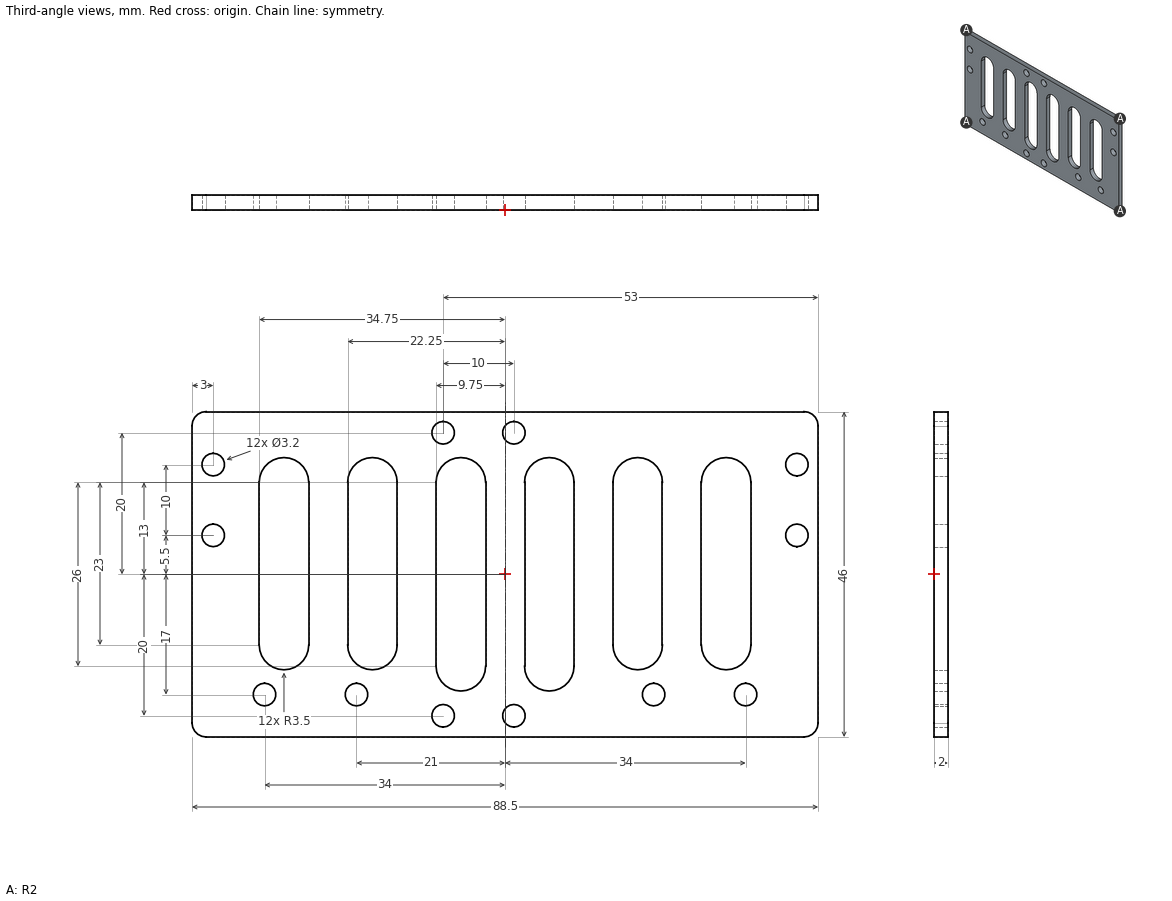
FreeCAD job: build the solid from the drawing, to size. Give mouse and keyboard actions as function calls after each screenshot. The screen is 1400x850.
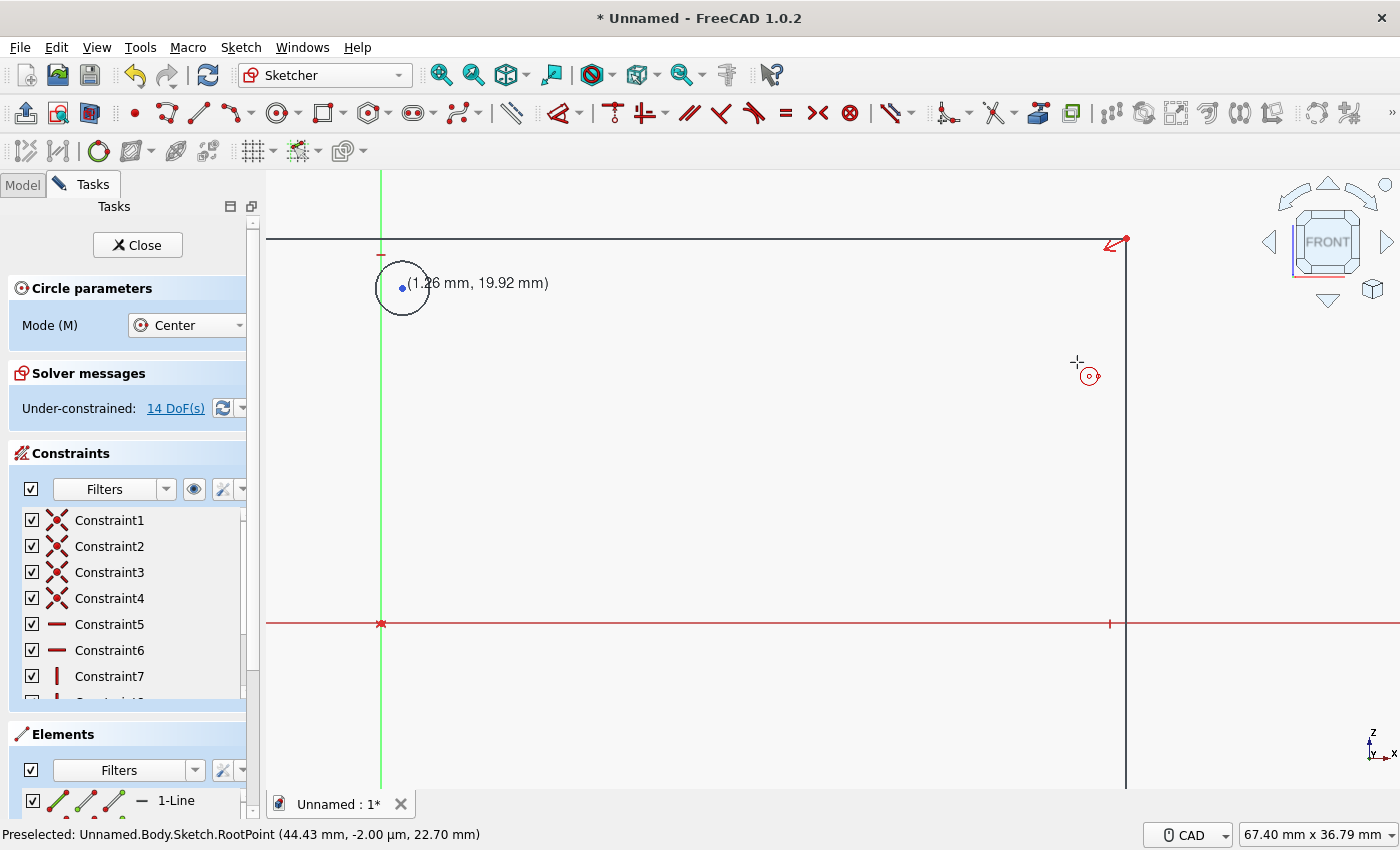
click(1075, 363)
click(1095, 344)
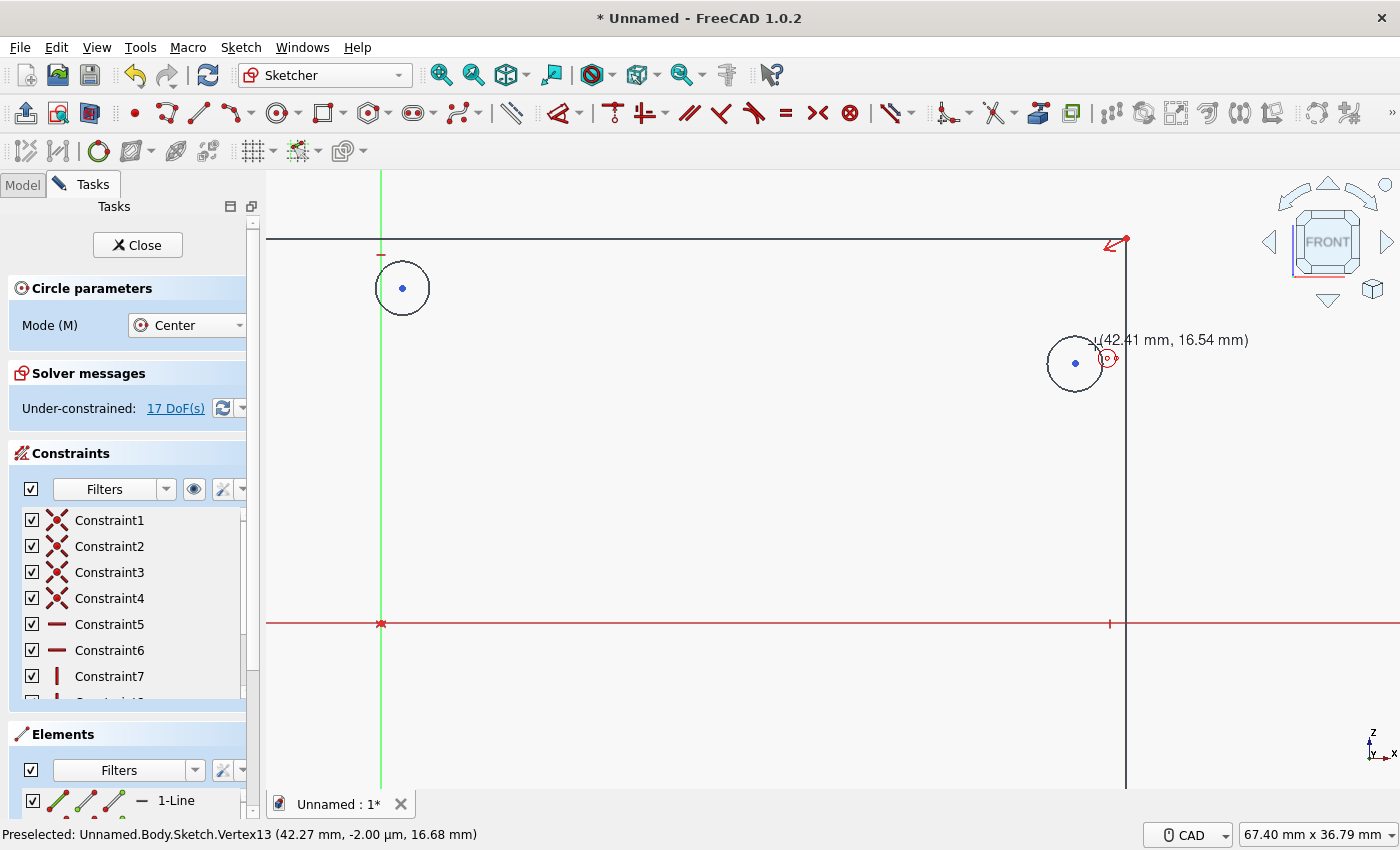
click(1075, 531)
click(1095, 512)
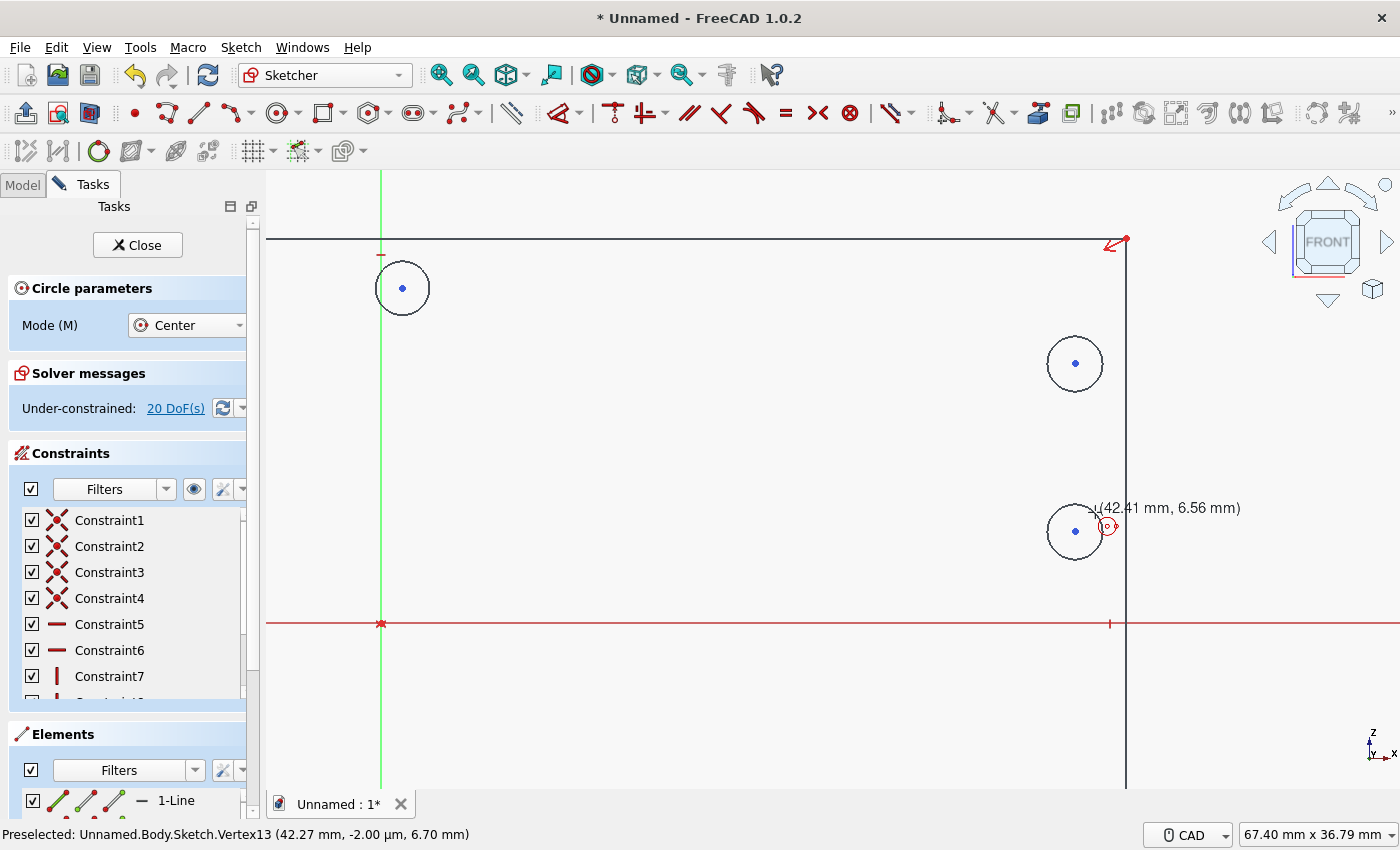
scroll(1077, 362, down, 4)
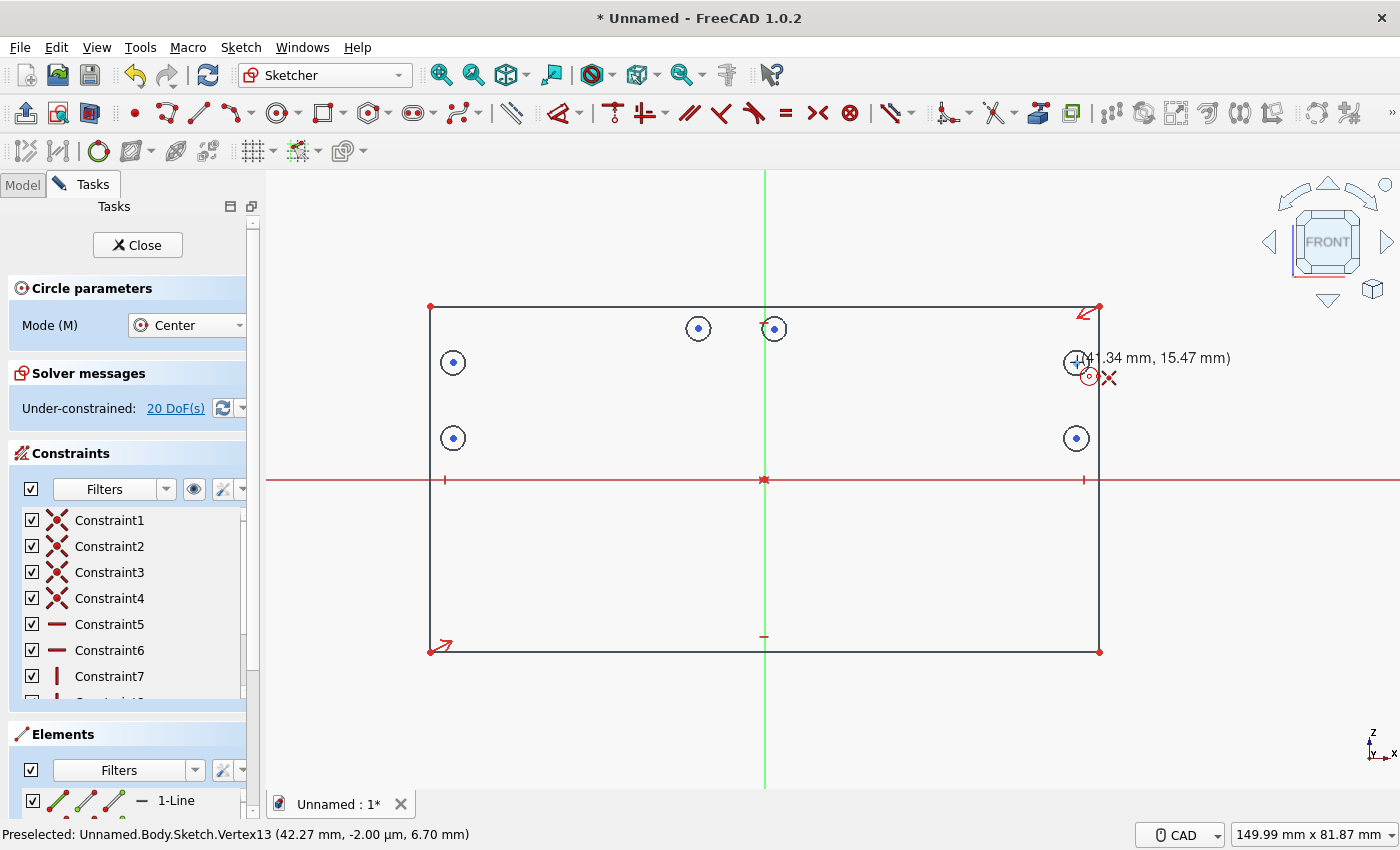
scroll(508, 608, up, 4)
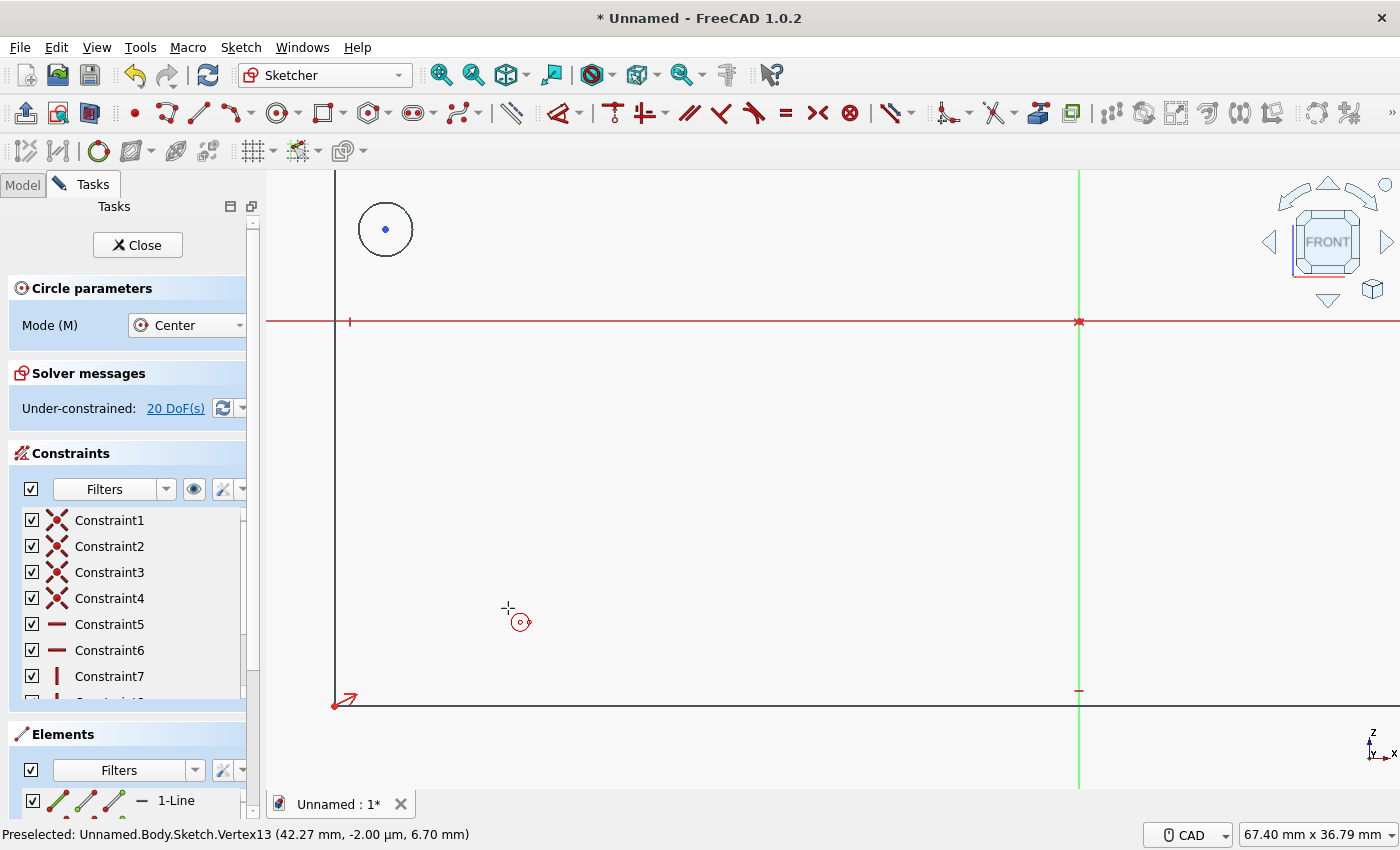
click(507, 607)
click(526, 588)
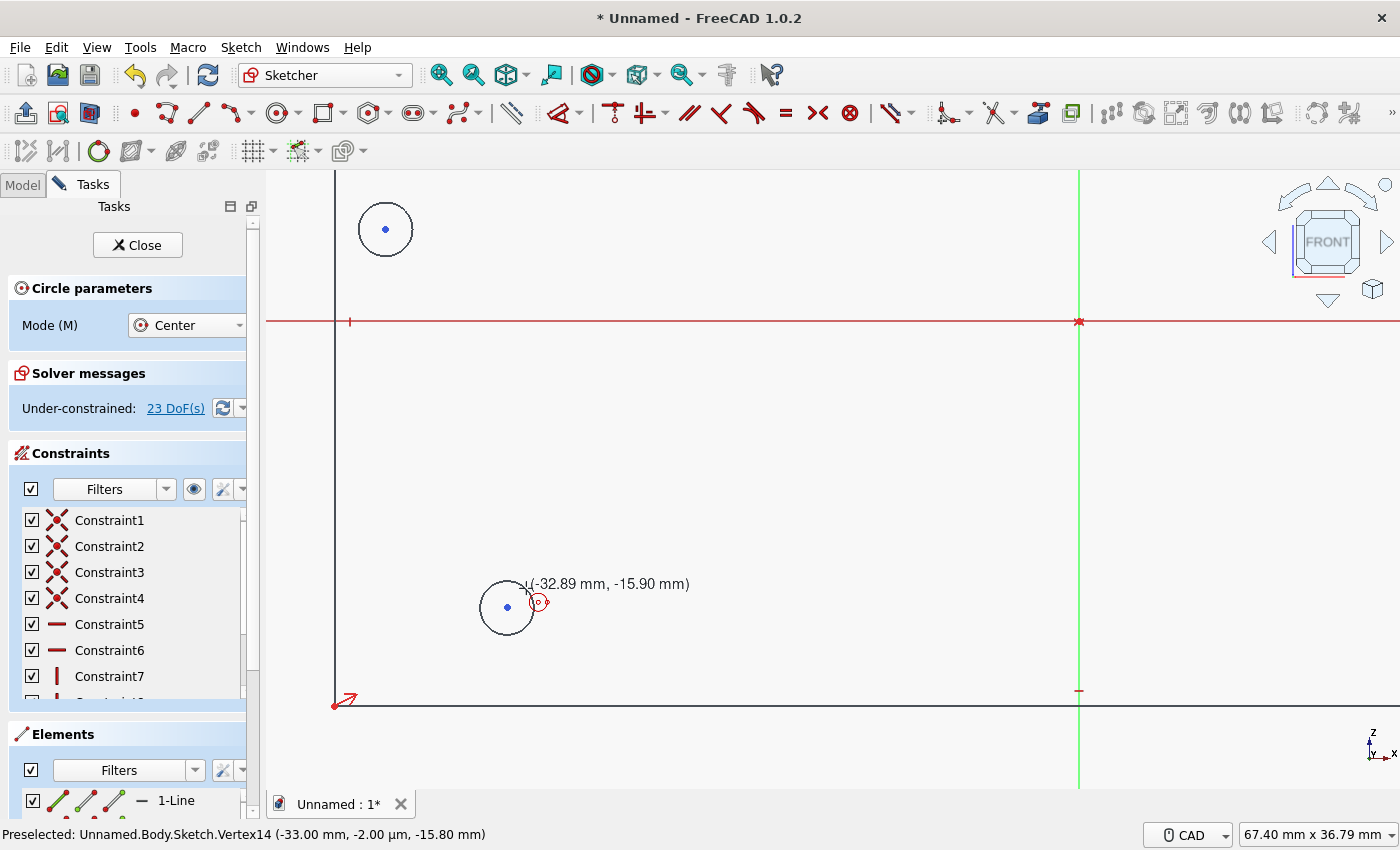
click(726, 607)
click(745, 588)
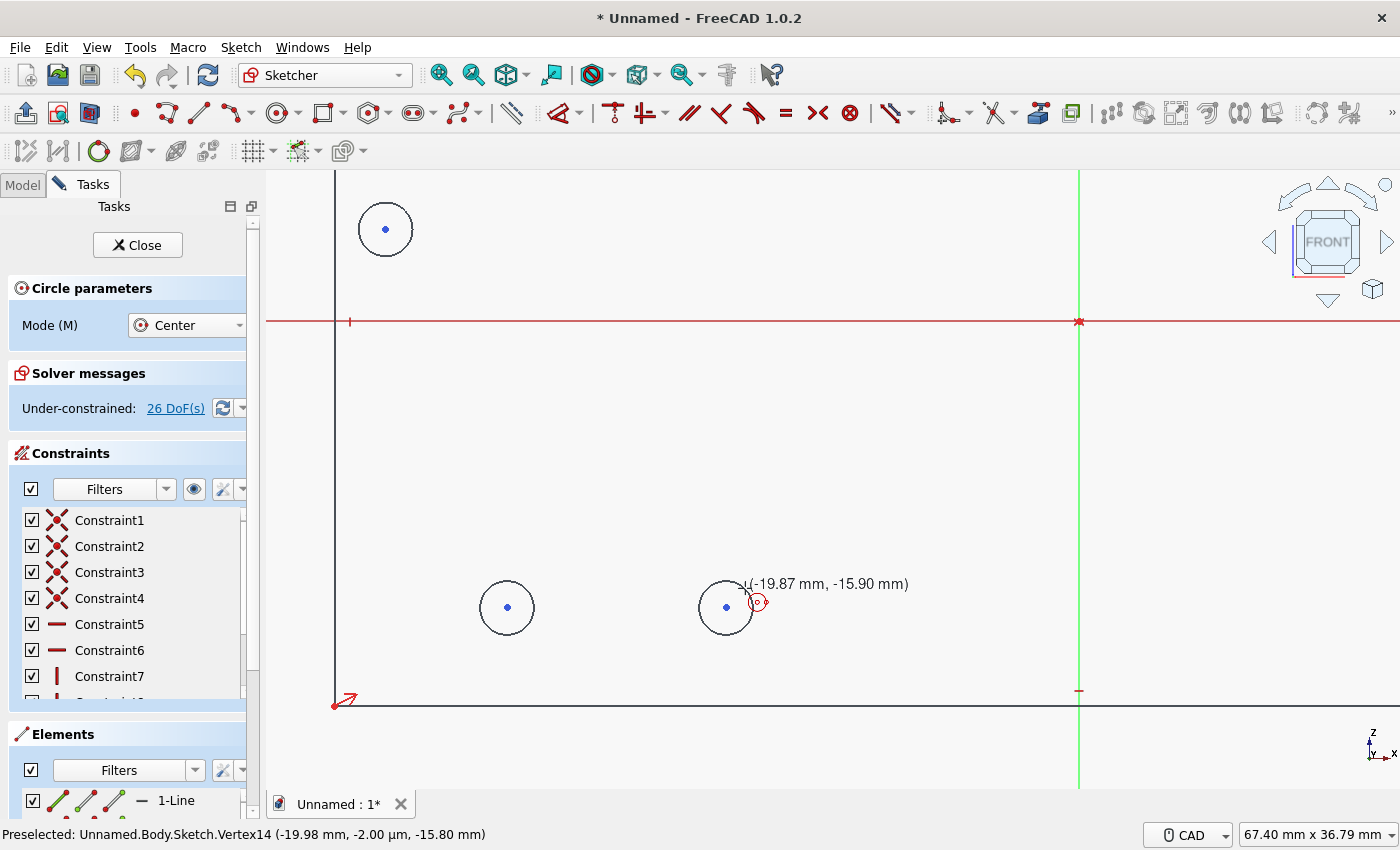
click(932, 658)
click(951, 639)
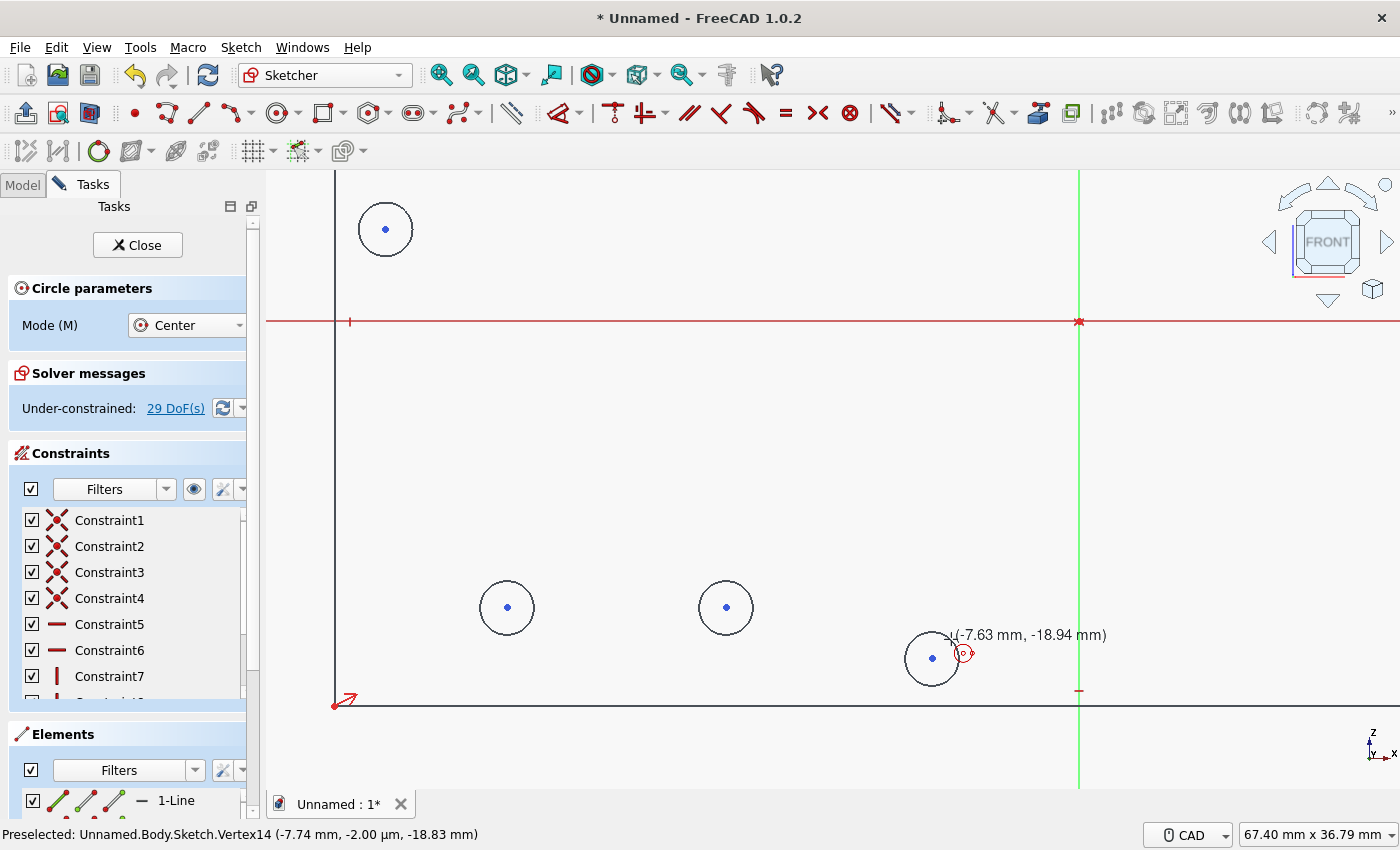
click(1100, 658)
click(1119, 639)